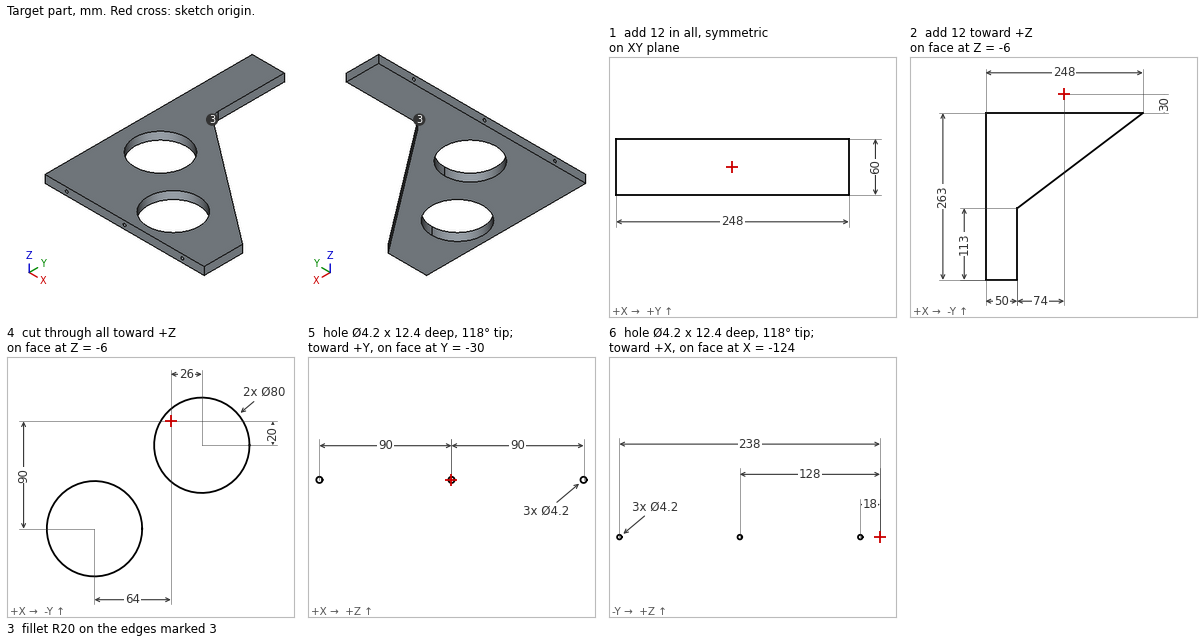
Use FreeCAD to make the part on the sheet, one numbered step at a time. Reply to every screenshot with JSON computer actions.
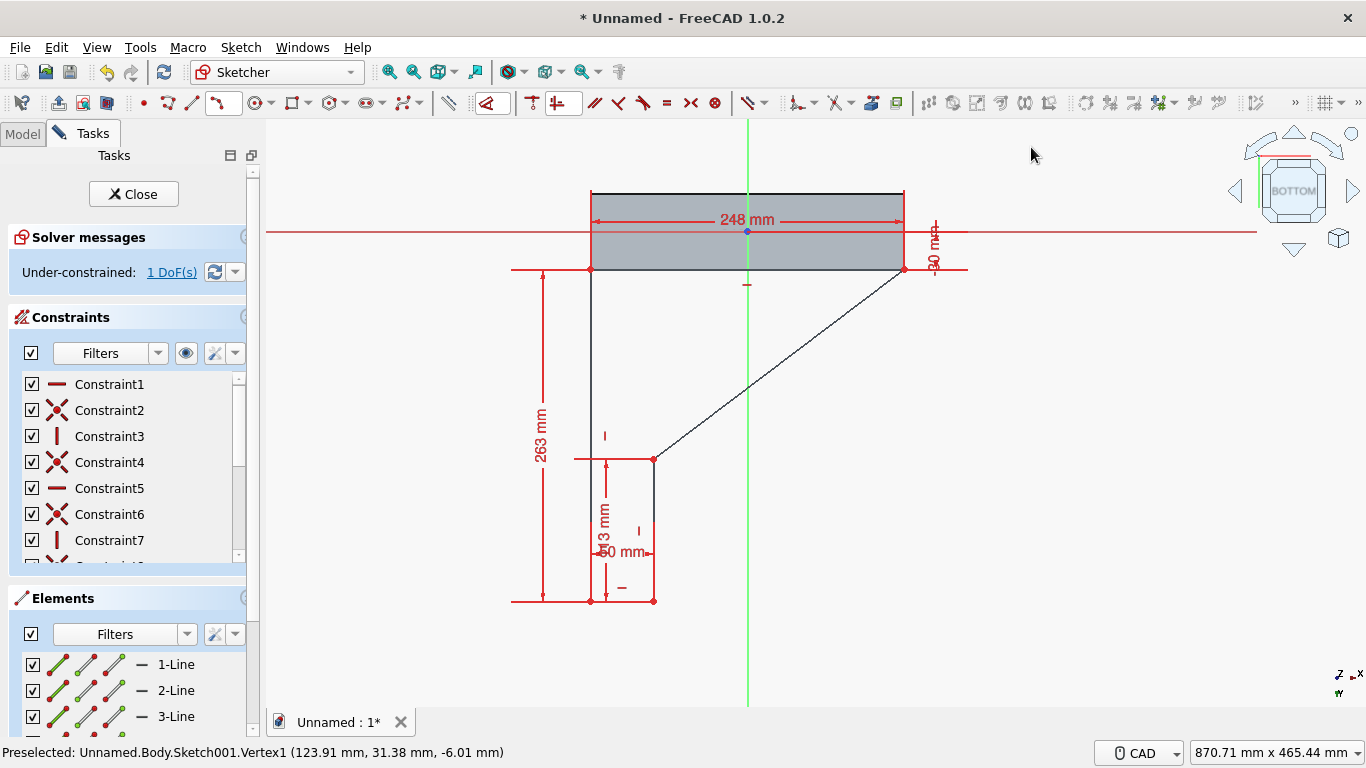
{"action": "left_click", "coordinate": [654, 602]}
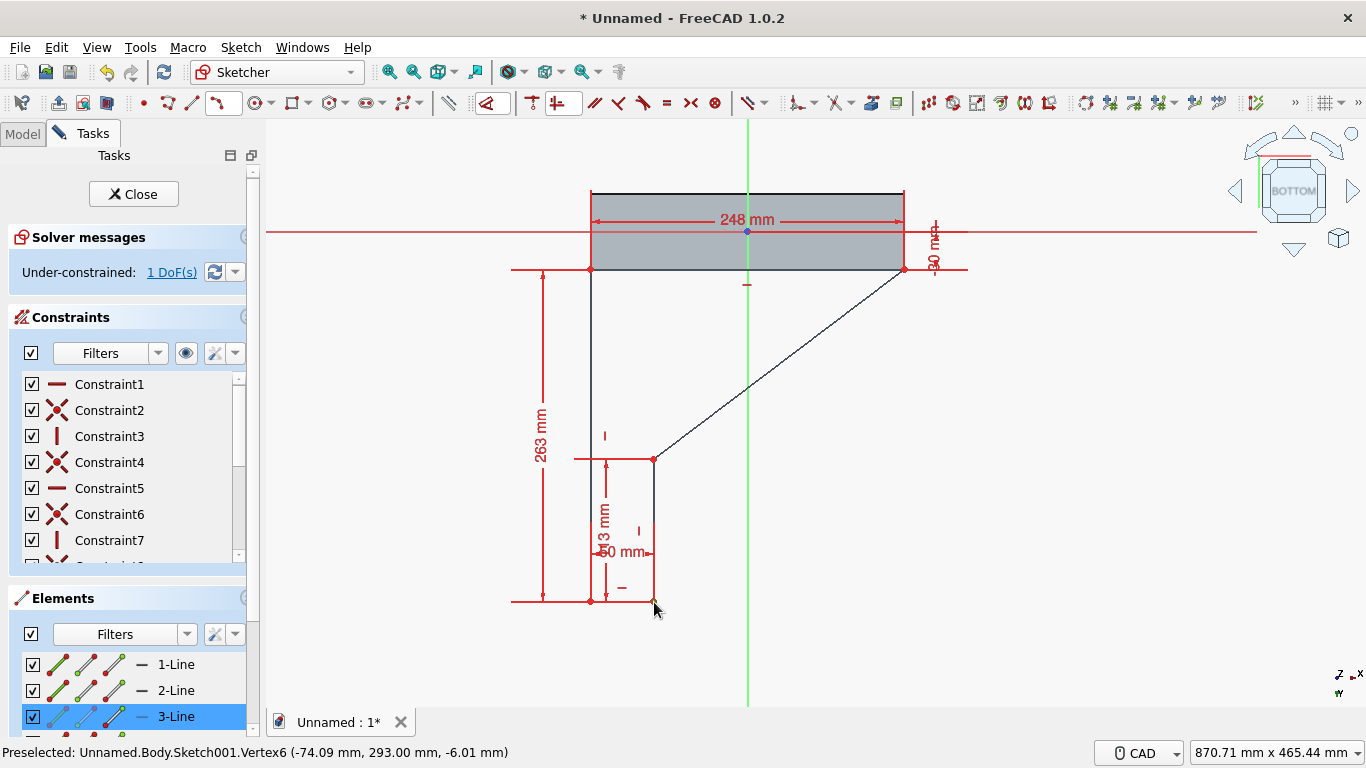
{"action": "key", "text": "l"}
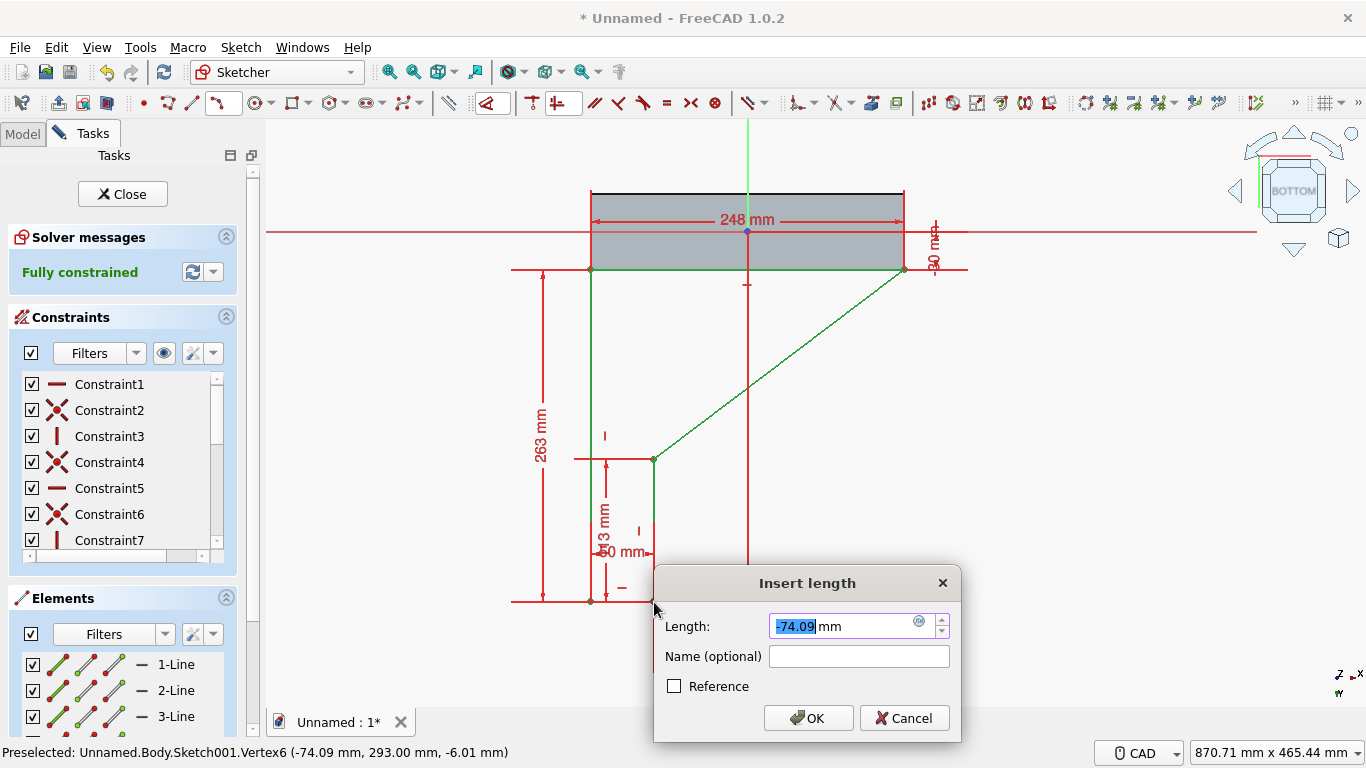
{"action": "type", "text": "-74"}
{"action": "key", "text": "Return"}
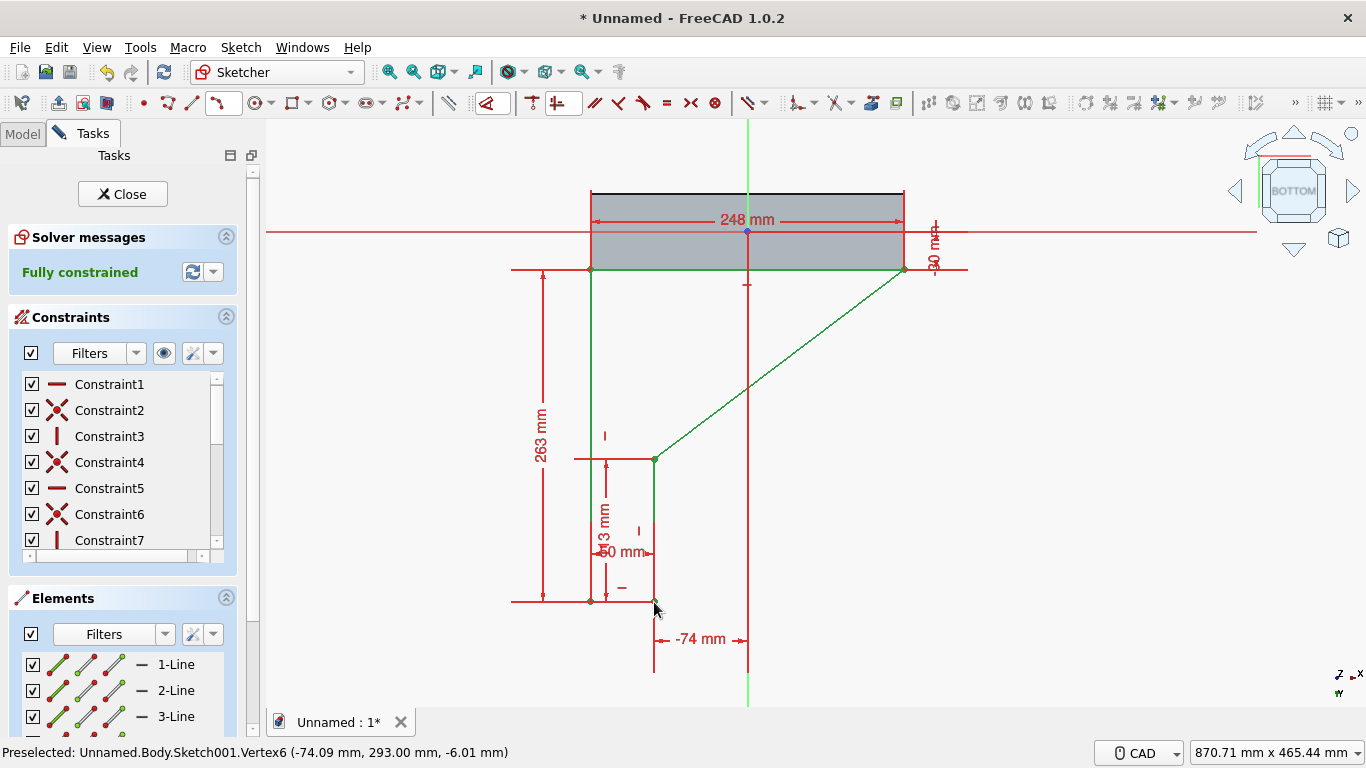
{"action": "left_click", "coordinate": [123, 194]}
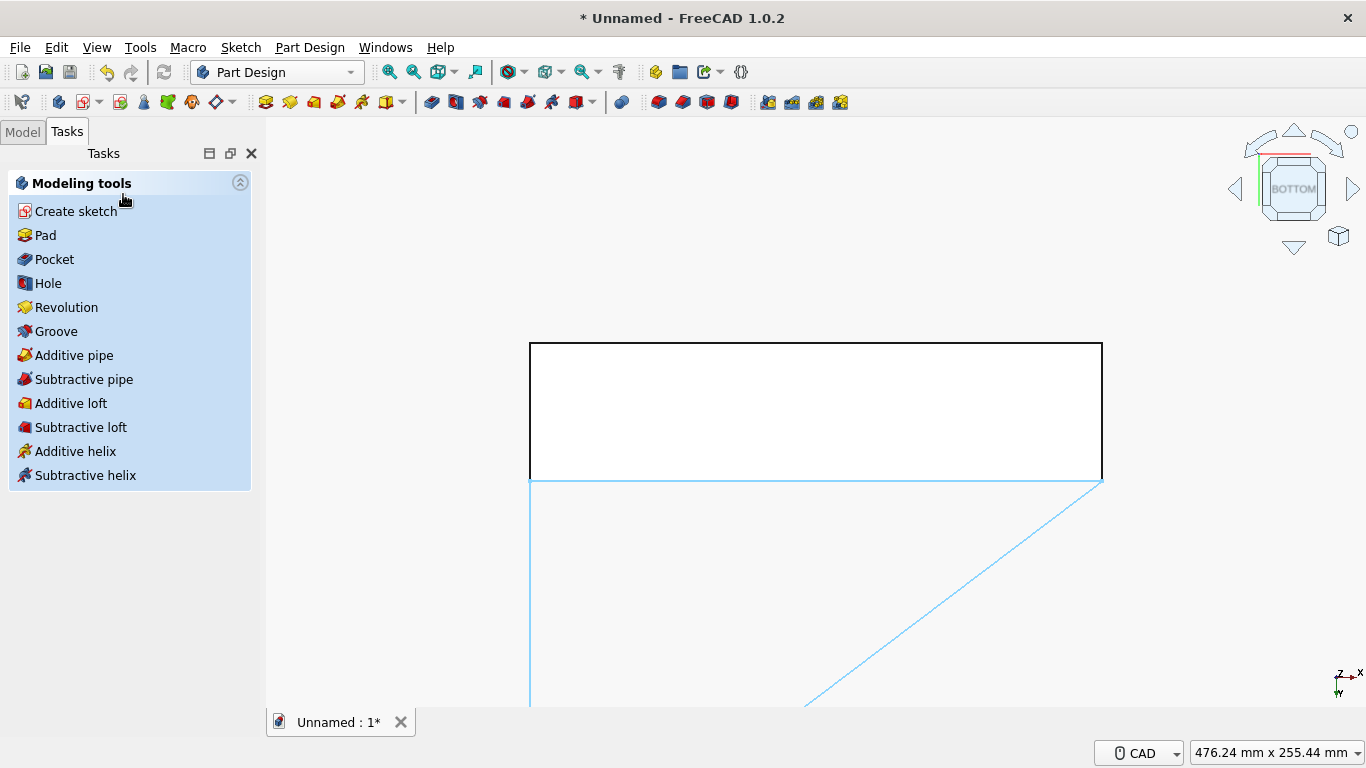
{"action": "left_click", "coordinate": [266, 102]}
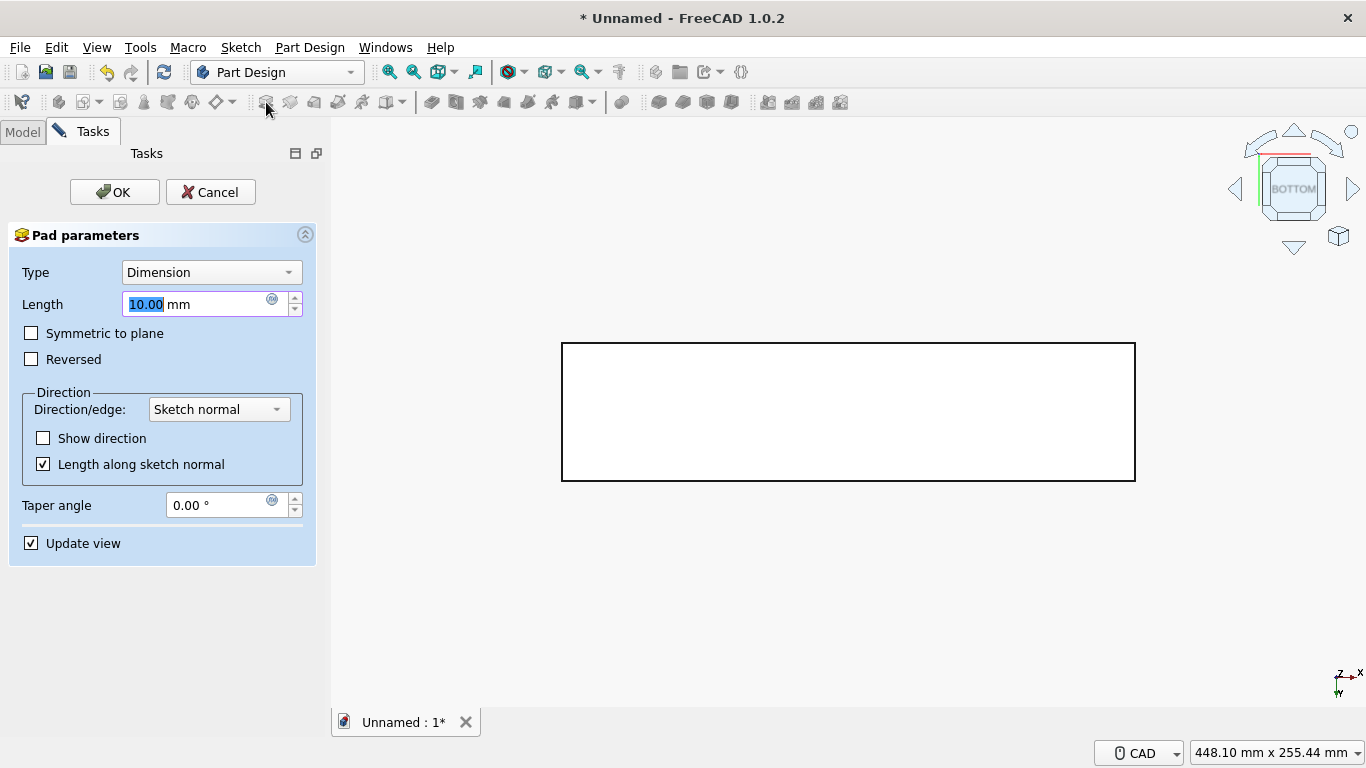
{"action": "type", "text": "12"}
{"action": "key", "text": "Tab"}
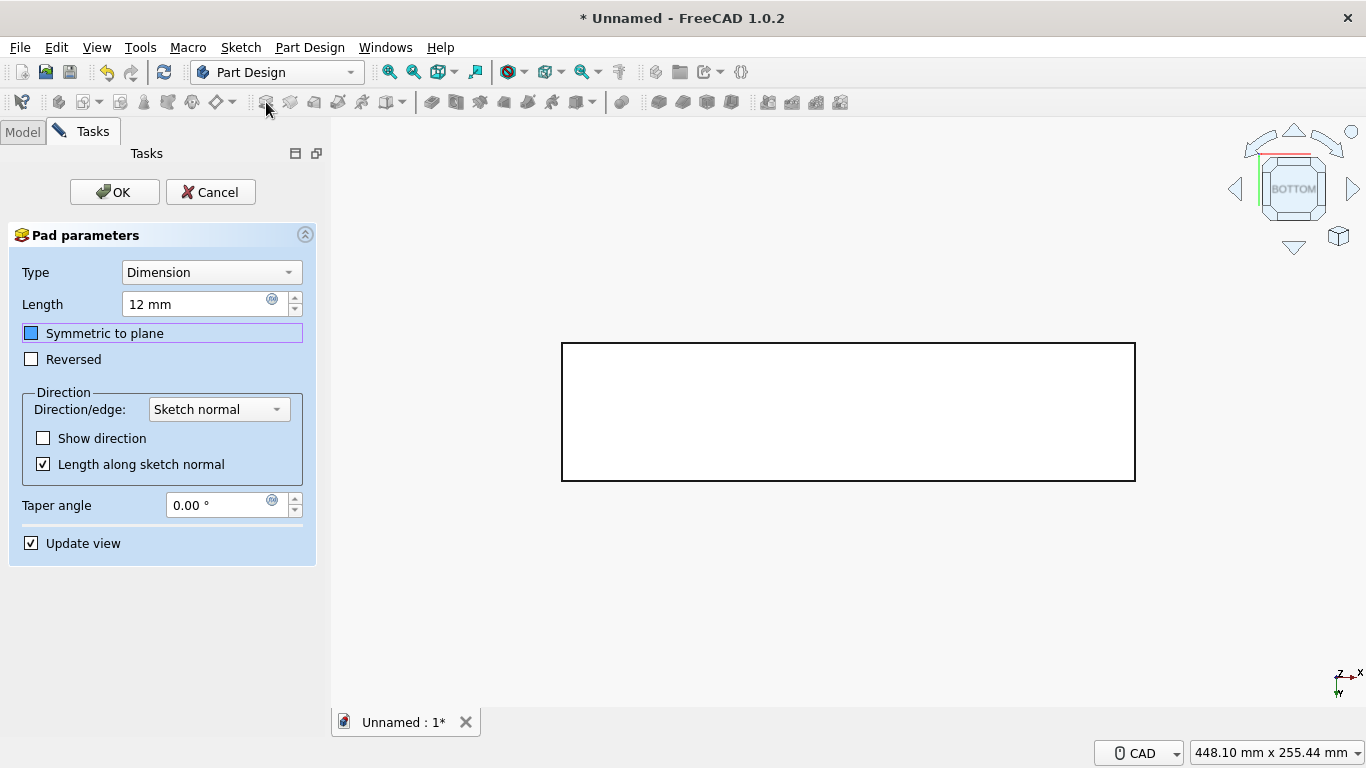
{"action": "left_click", "coordinate": [30, 359]}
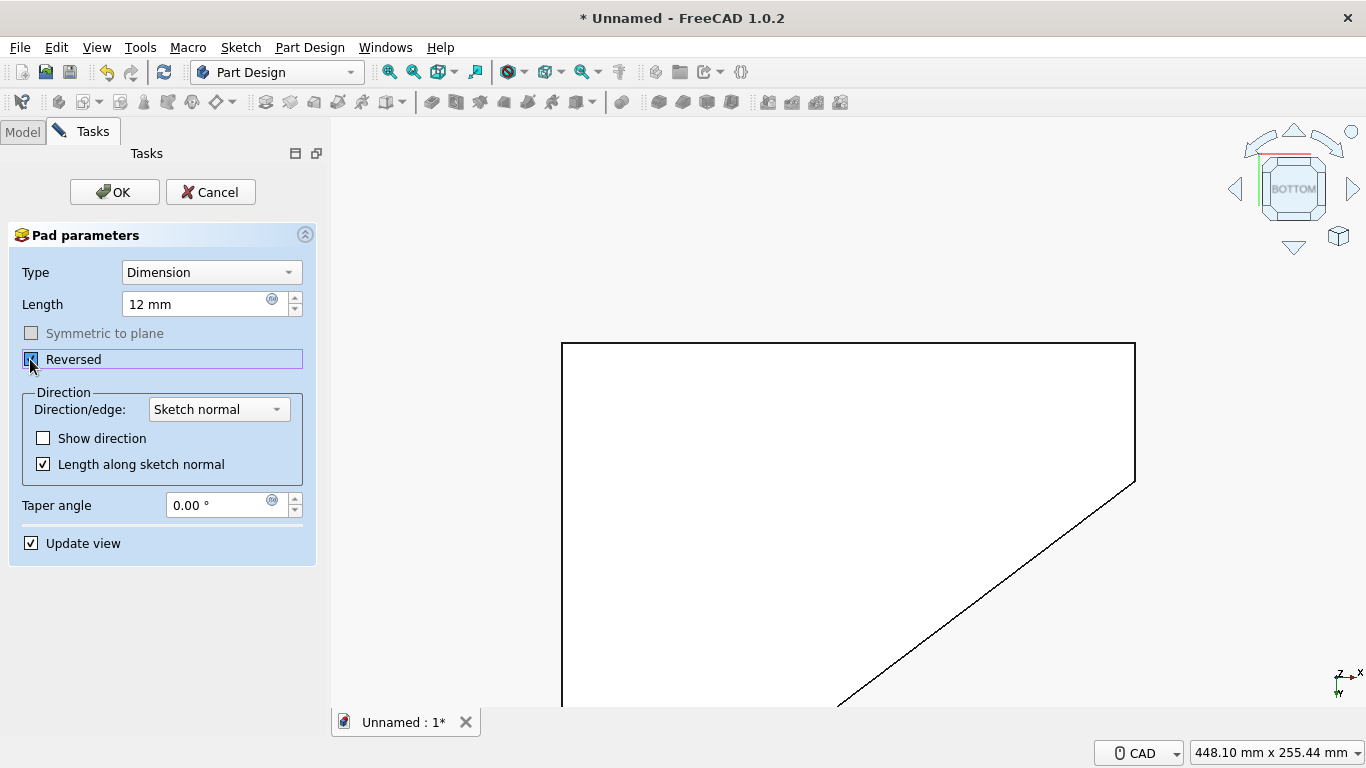
{"action": "left_click", "coordinate": [115, 192]}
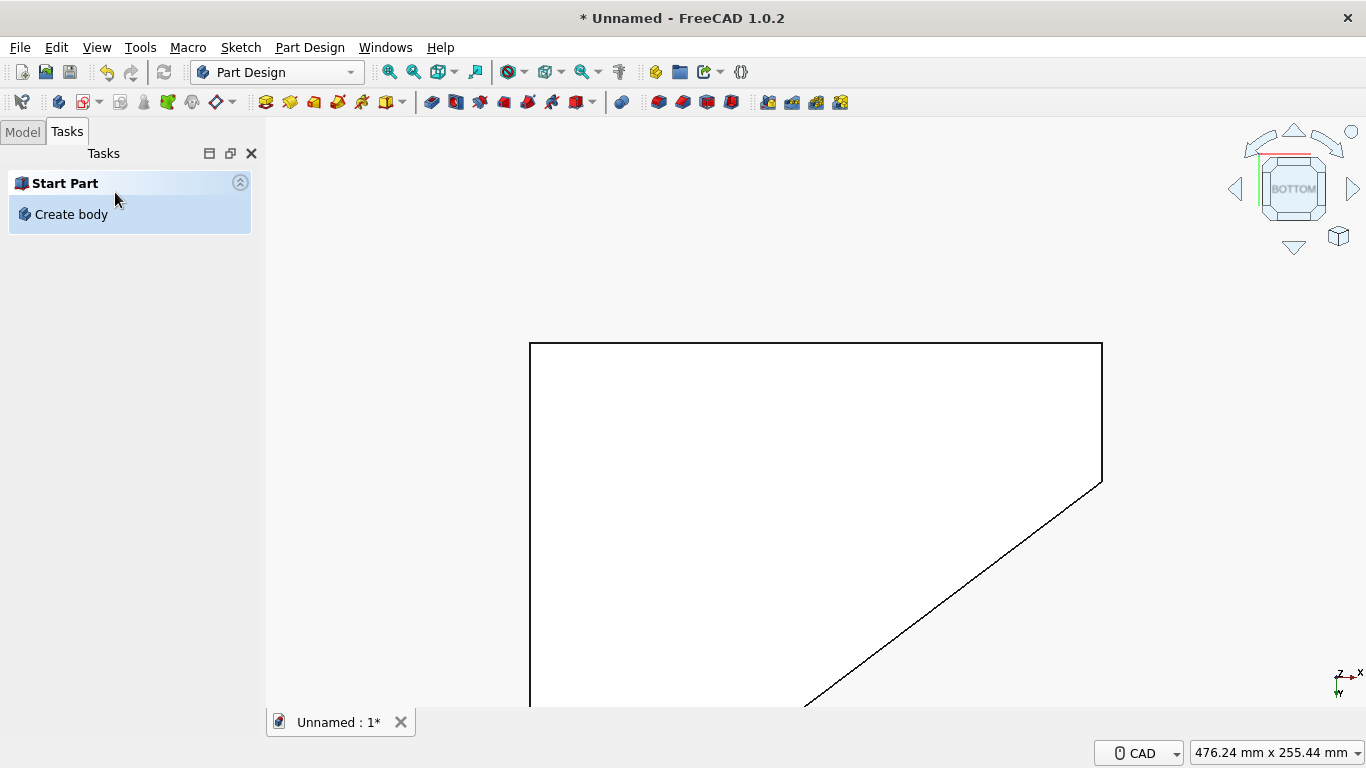
{"action": "key", "text": "v f"}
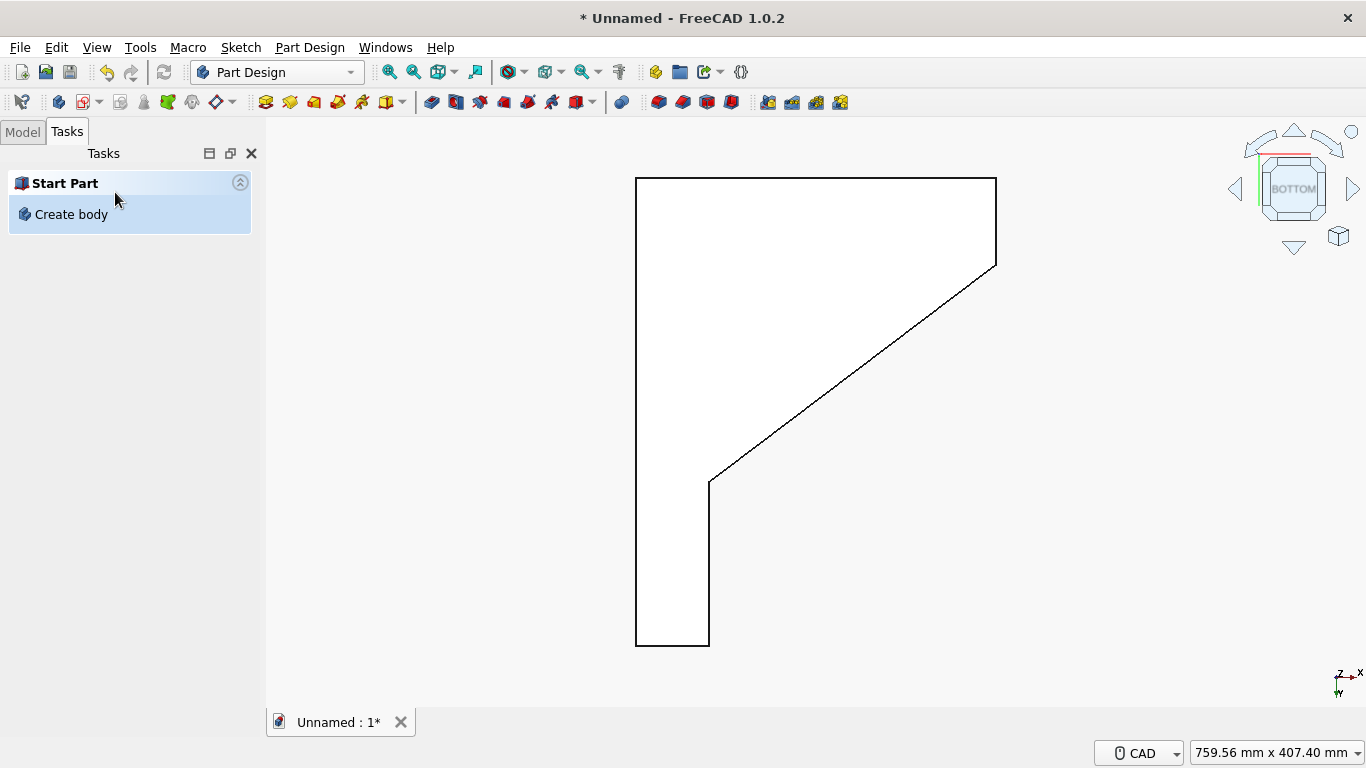
{"action": "scroll", "coordinate": [709, 481], "scroll_direction": "up", "scroll_amount": 5}